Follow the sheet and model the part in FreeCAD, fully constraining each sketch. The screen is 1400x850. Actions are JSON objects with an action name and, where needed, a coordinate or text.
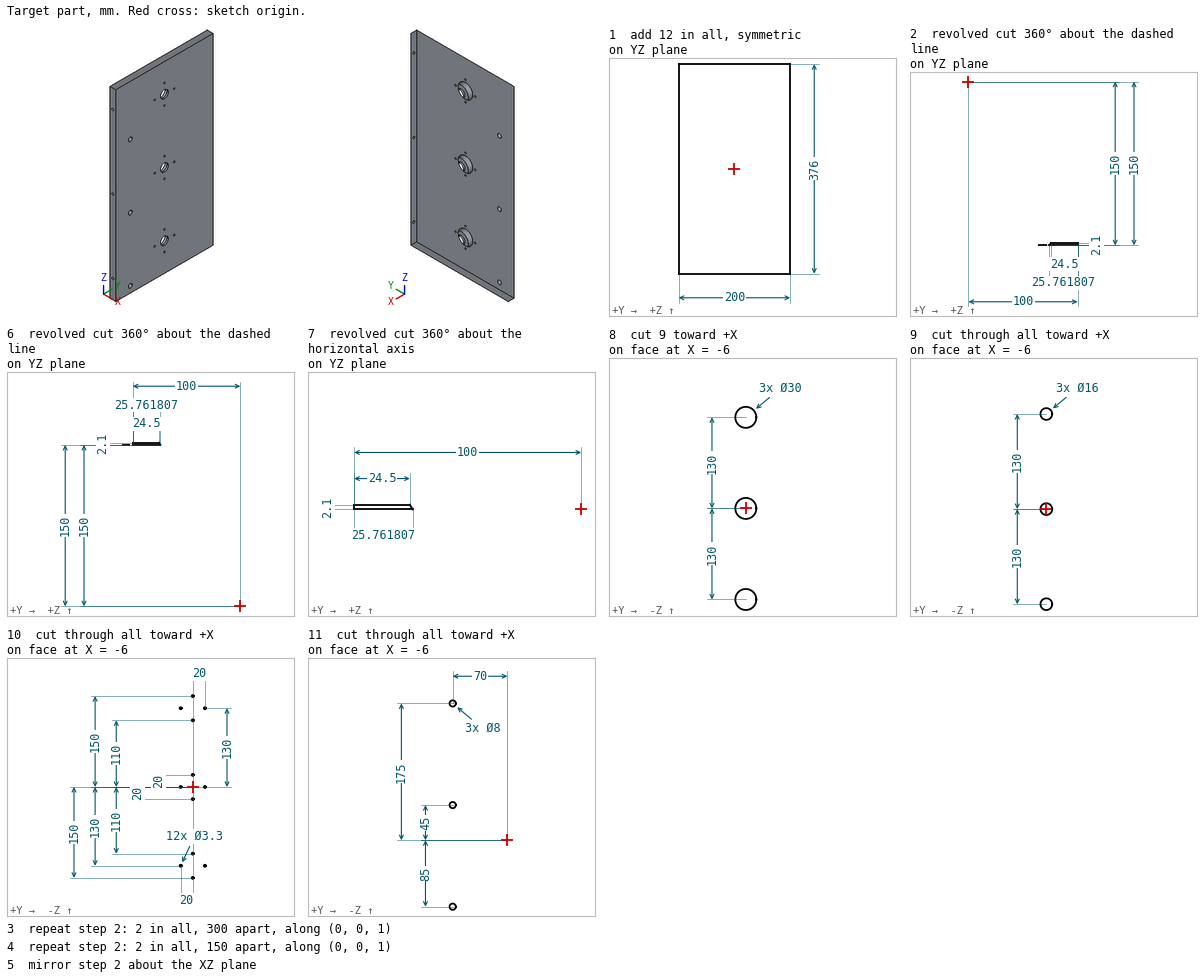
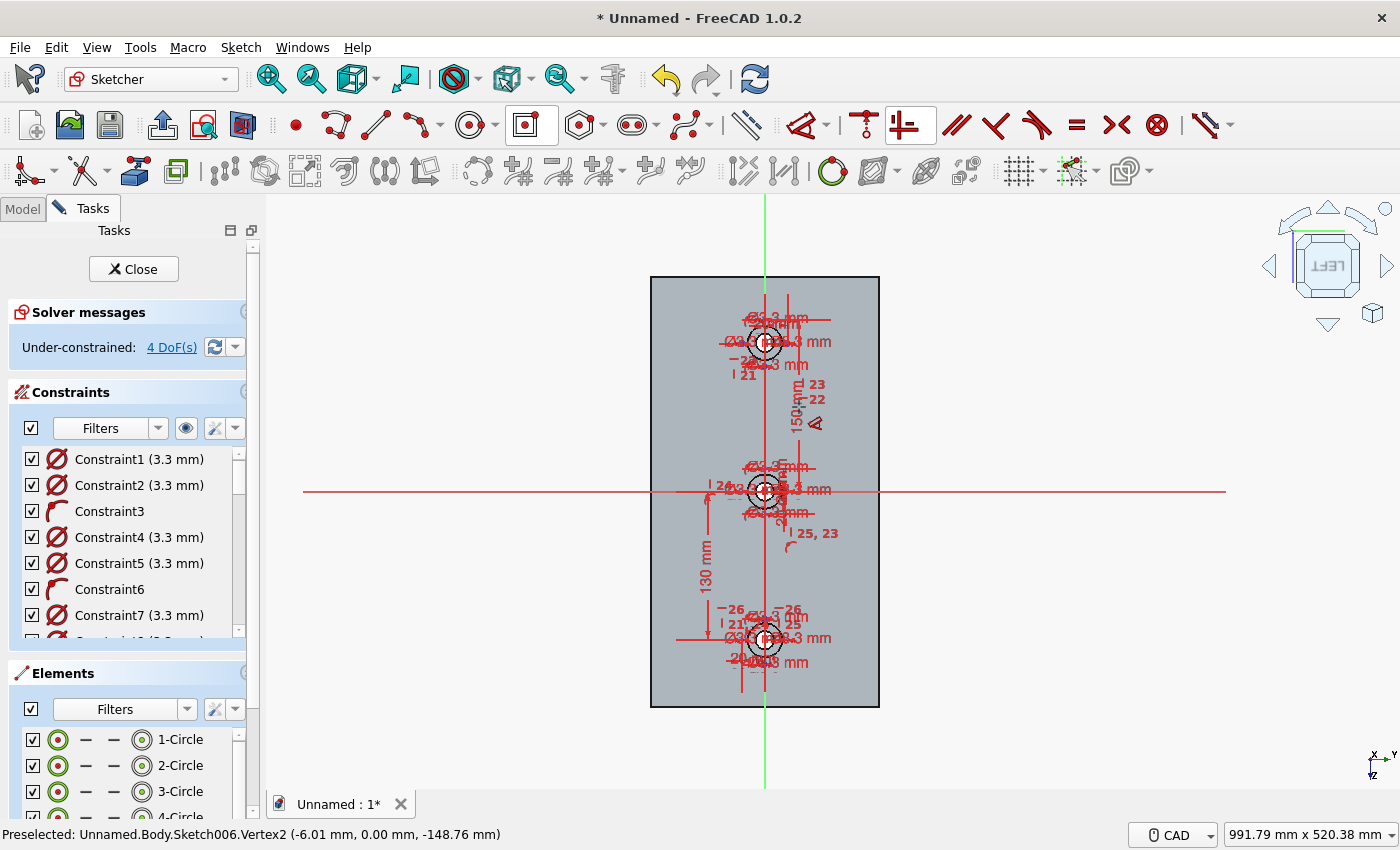
{"action": "left_click", "coordinate": [788, 344]}
{"action": "left_click", "coordinate": [822, 384]}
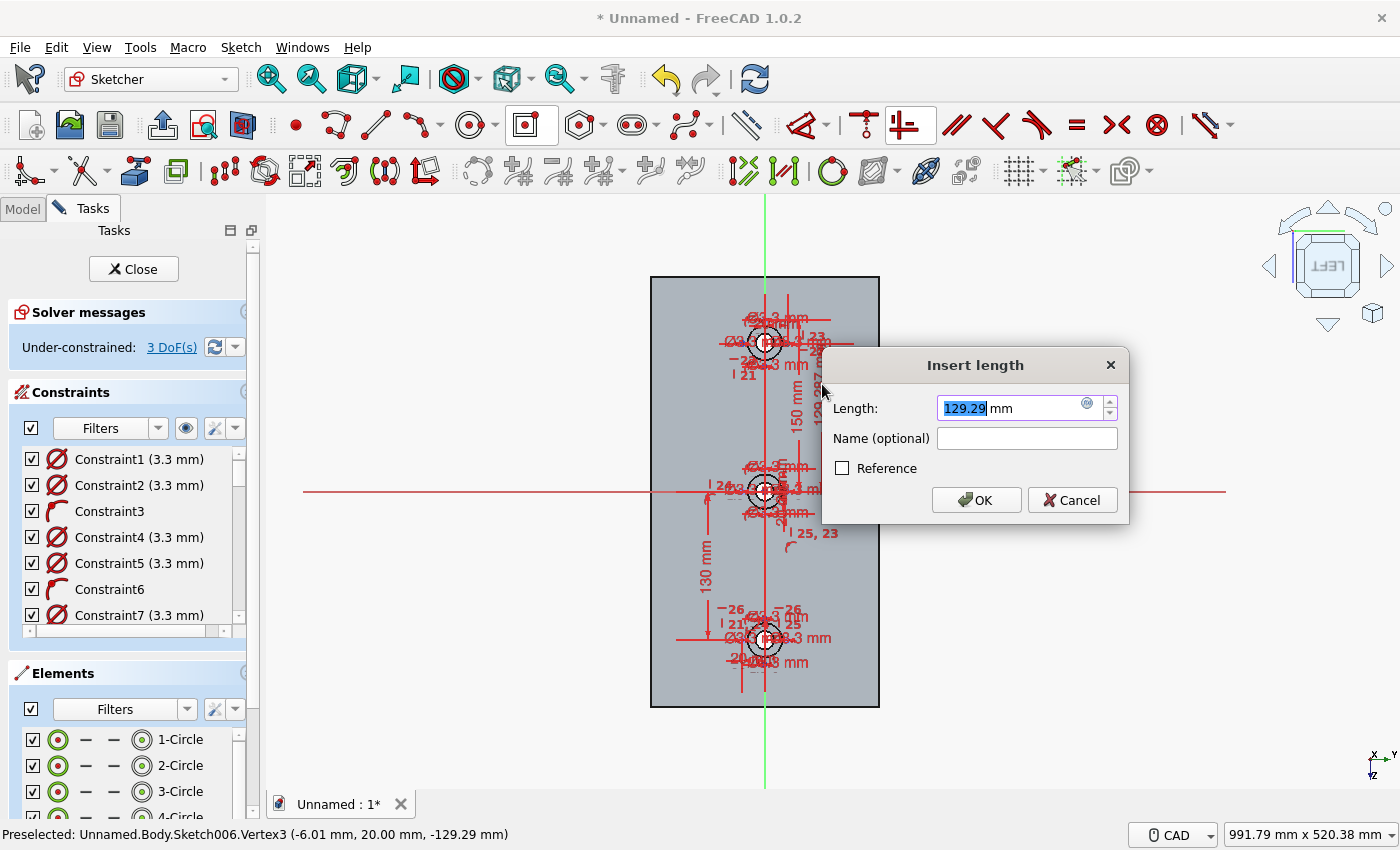
{"action": "type", "text": "130"}
{"action": "key", "text": "Return"}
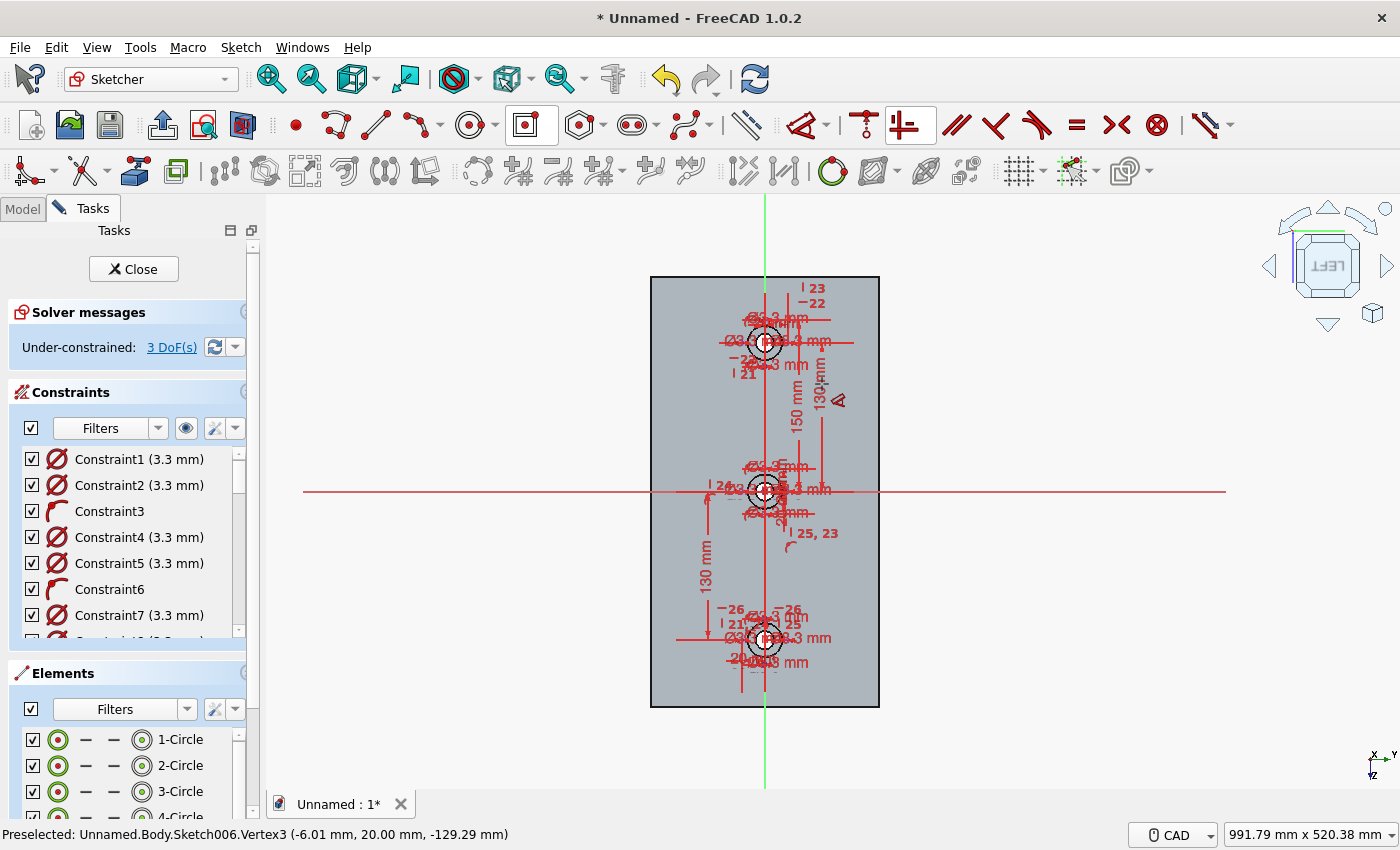
{"action": "left_click", "coordinate": [765, 367]}
{"action": "left_click", "coordinate": [799, 429]}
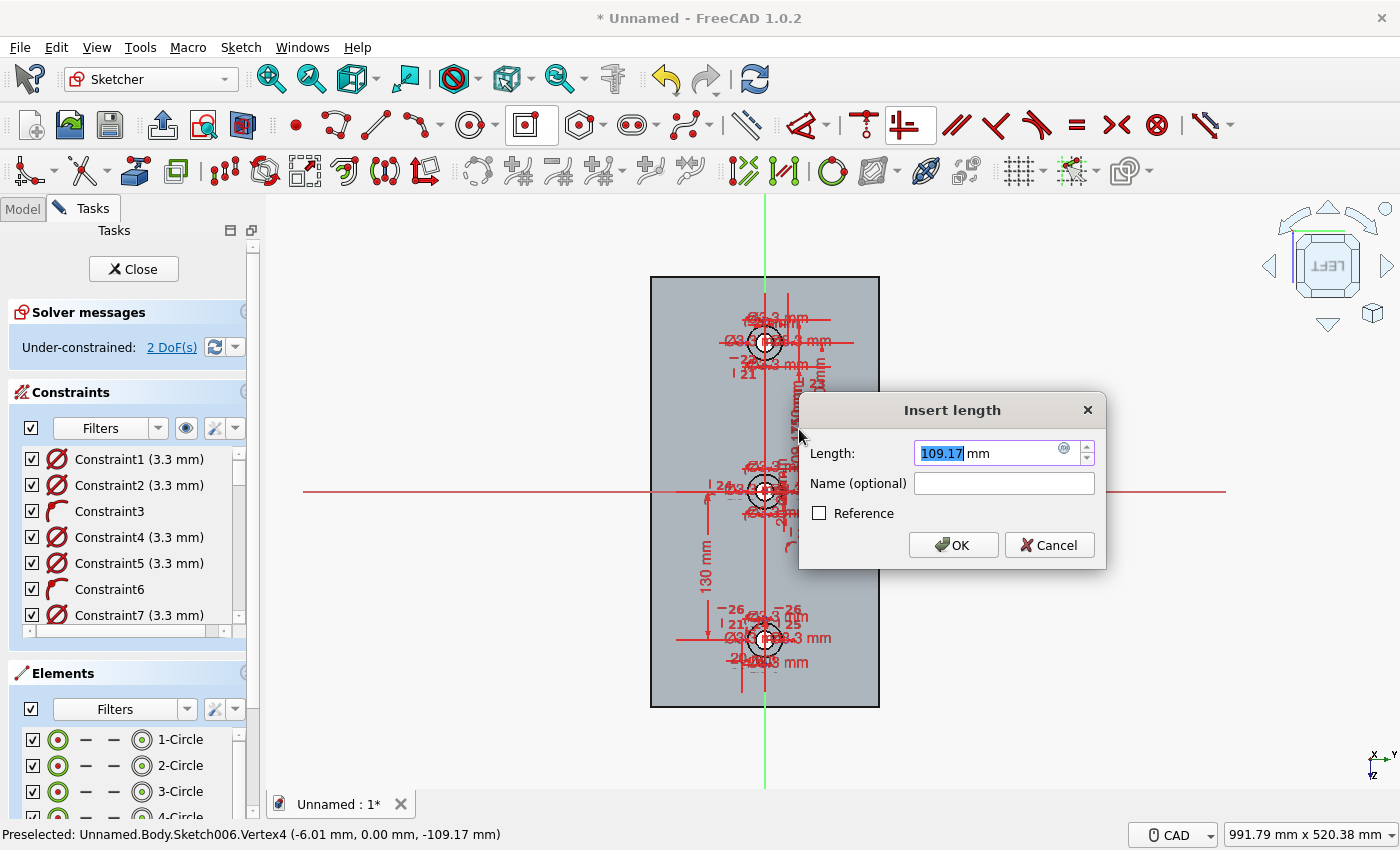
{"action": "type", "text": "110"}
{"action": "key", "text": "Return"}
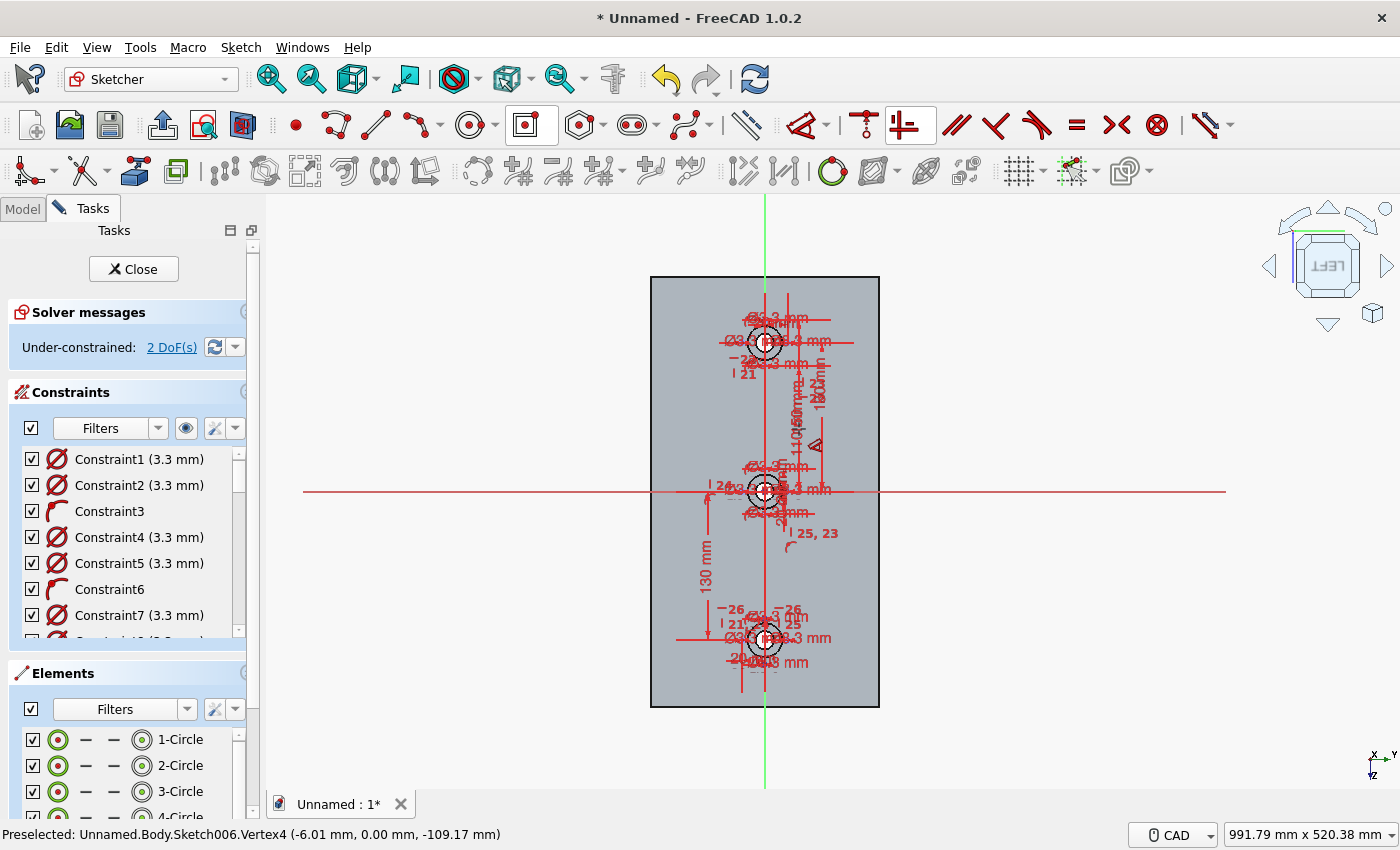
{"action": "left_click", "coordinate": [765, 619]}
{"action": "left_click", "coordinate": [799, 555]}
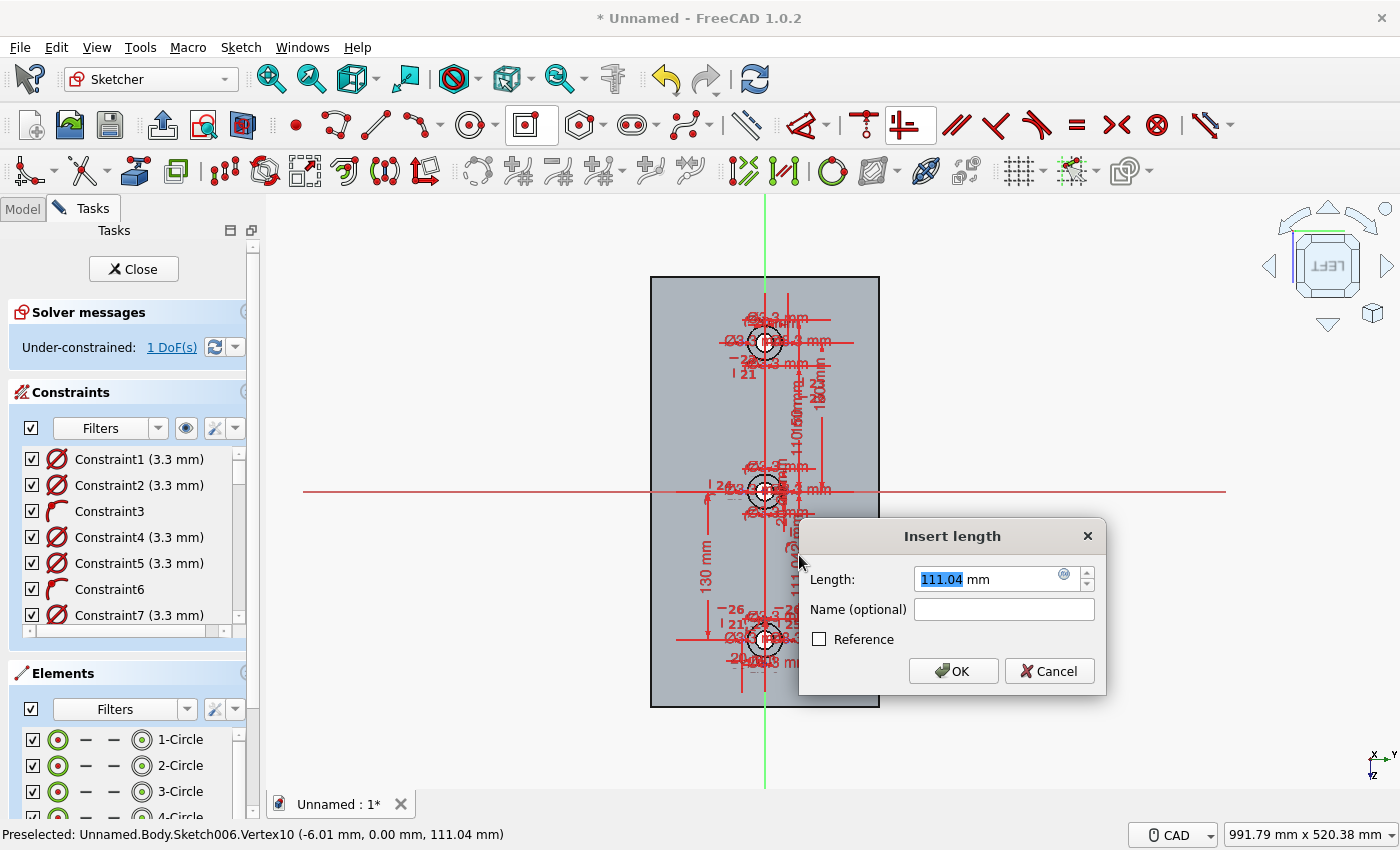
{"action": "type", "text": "110"}
{"action": "key", "text": "Return"}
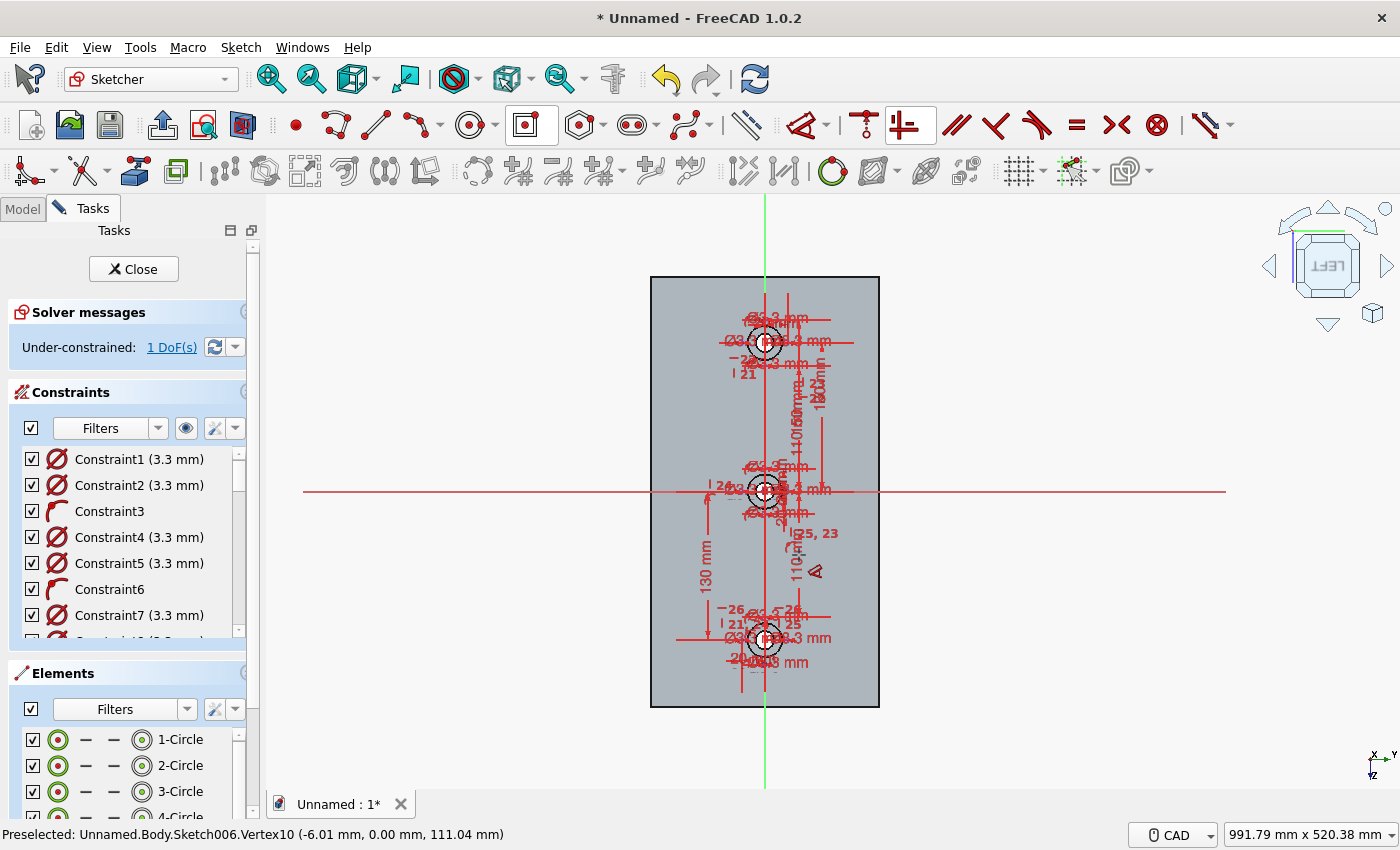
{"action": "left_click", "coordinate": [765, 665]}
{"action": "left_click", "coordinate": [799, 578]}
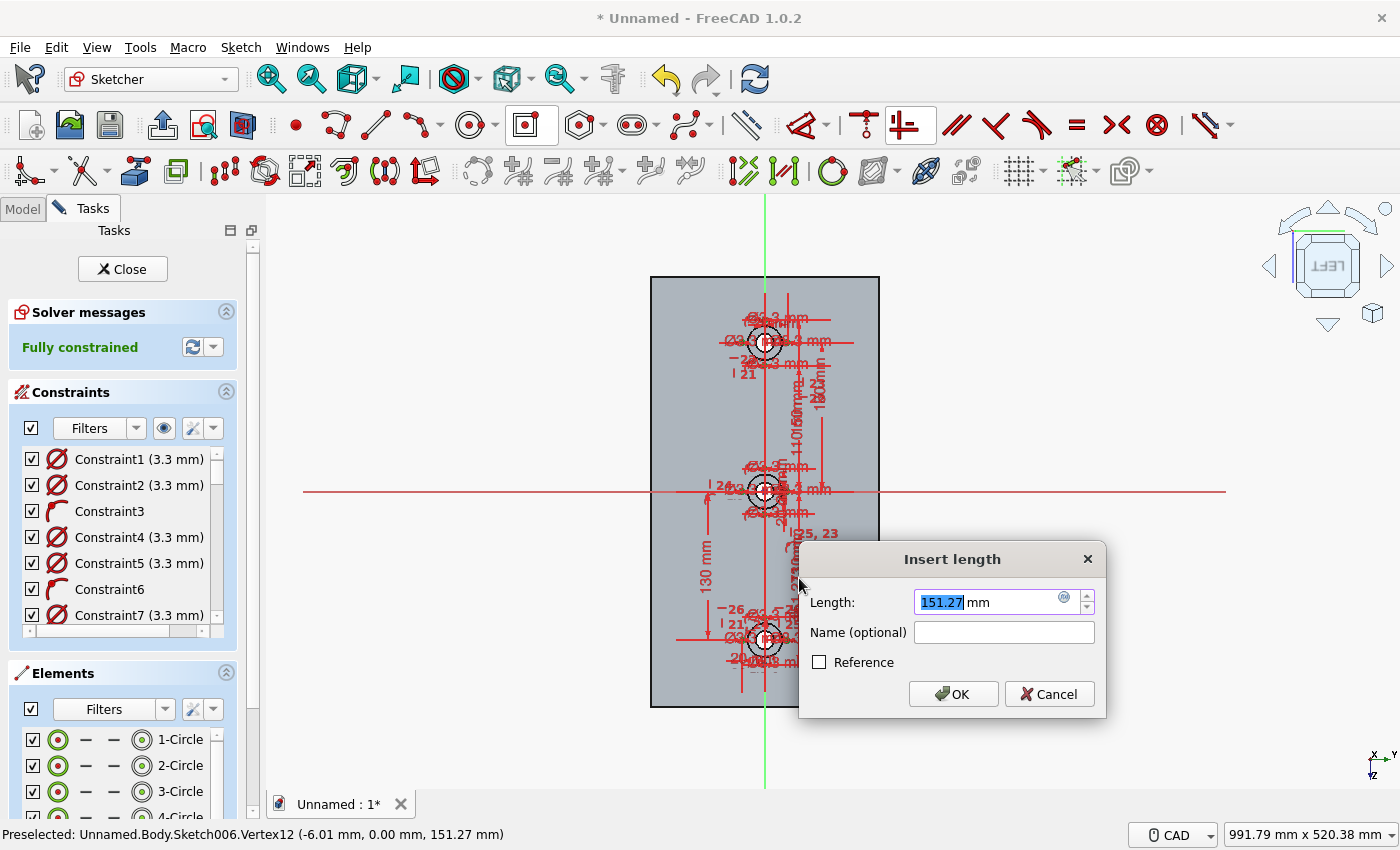
{"action": "type", "text": "150"}
{"action": "key", "text": "Return"}
{"action": "key", "text": "Escape"}